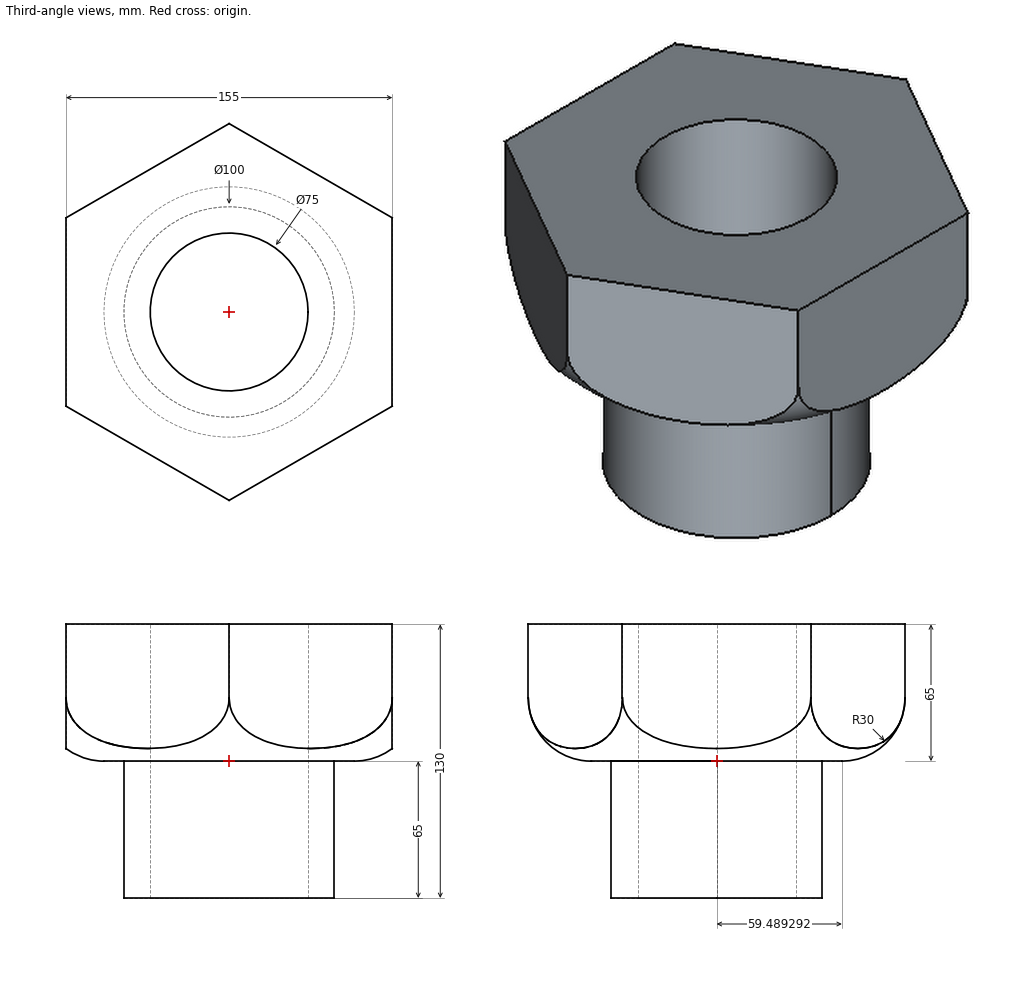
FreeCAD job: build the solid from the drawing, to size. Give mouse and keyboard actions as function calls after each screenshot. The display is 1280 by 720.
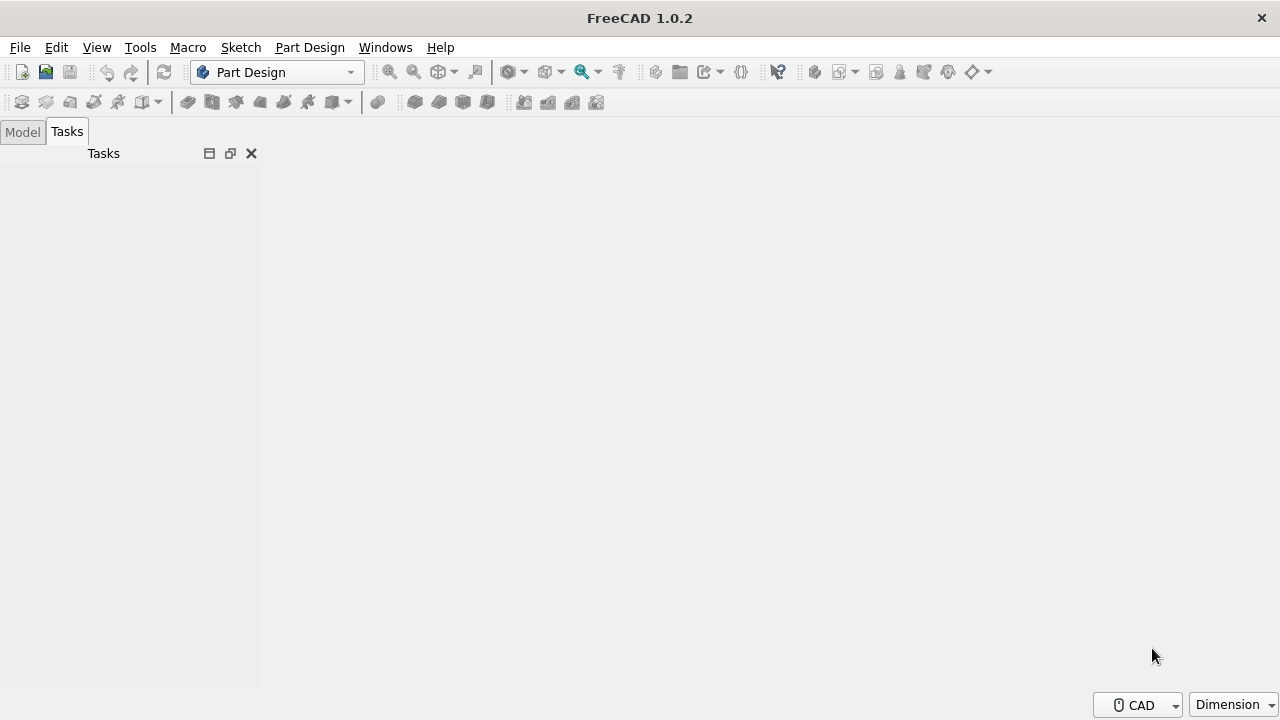
key(ctrl+n)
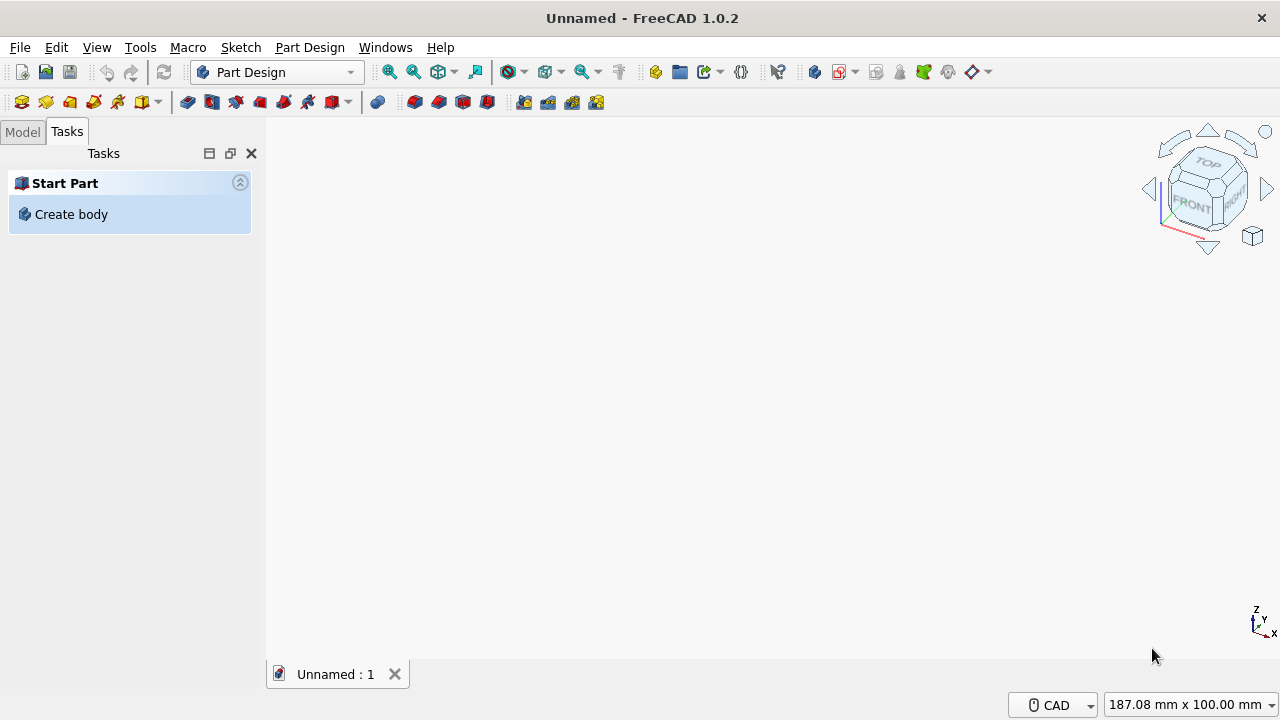
click(840, 72)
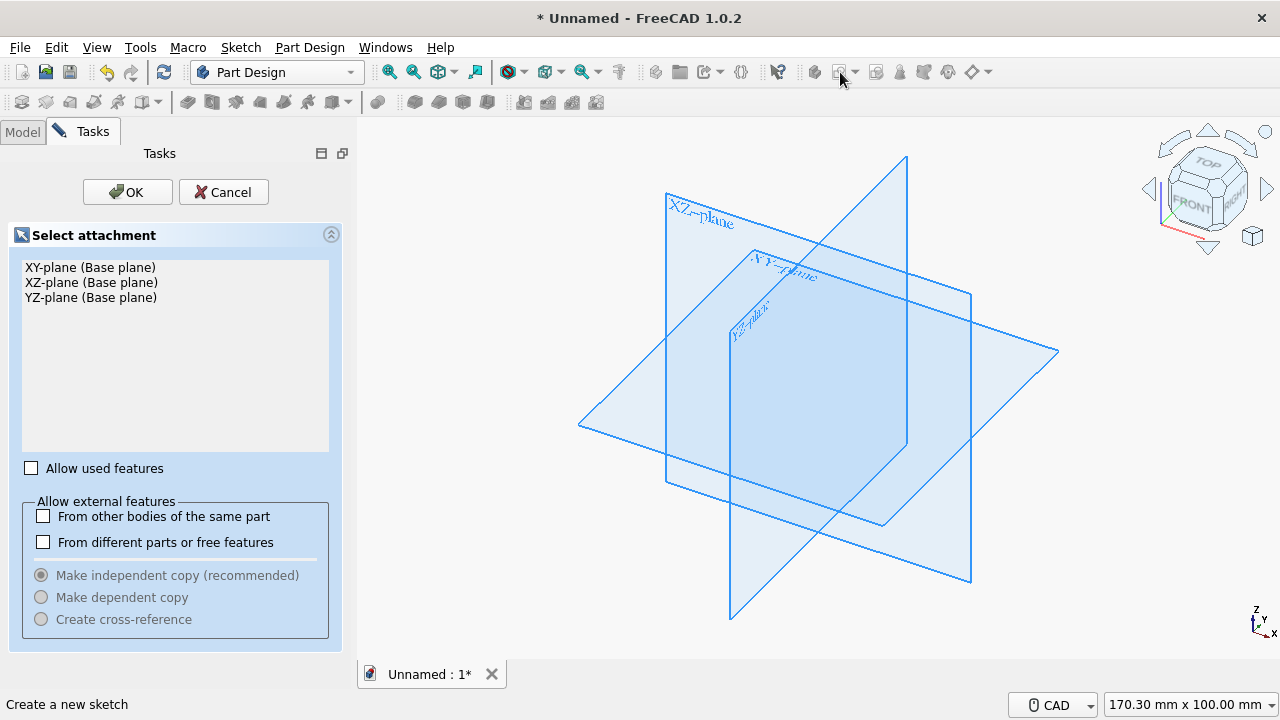
click(82, 268)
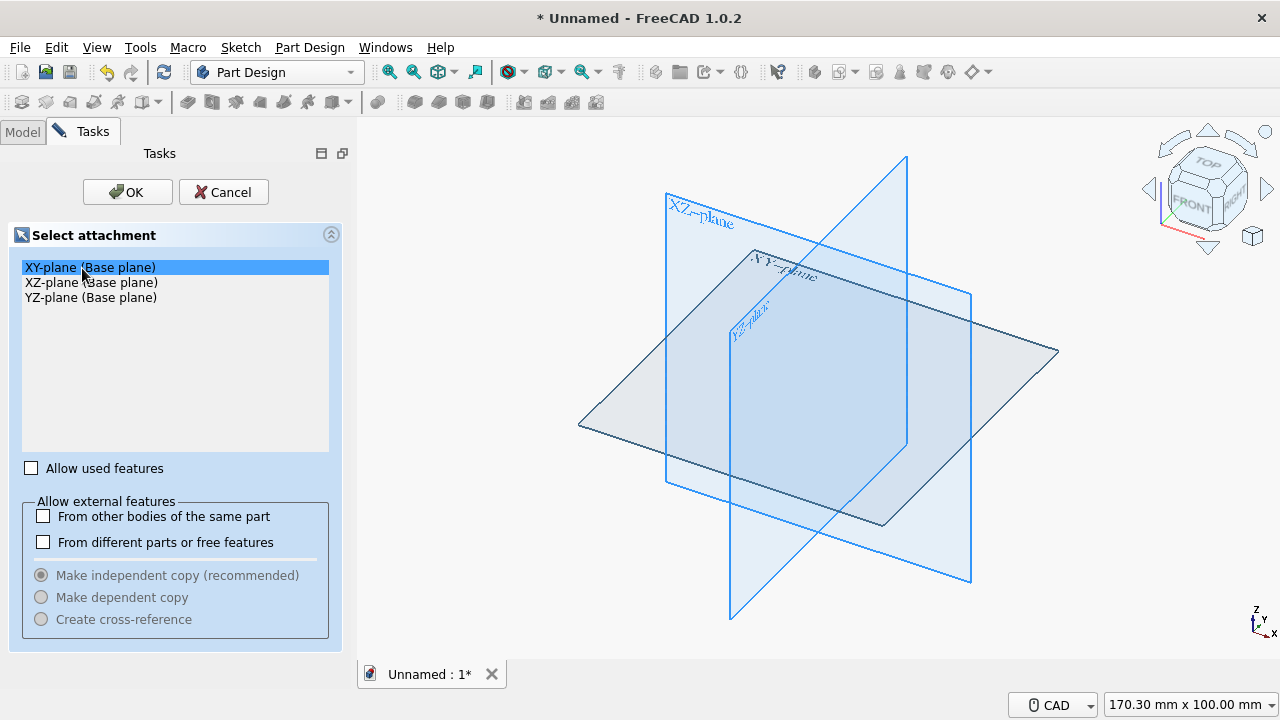
click(128, 192)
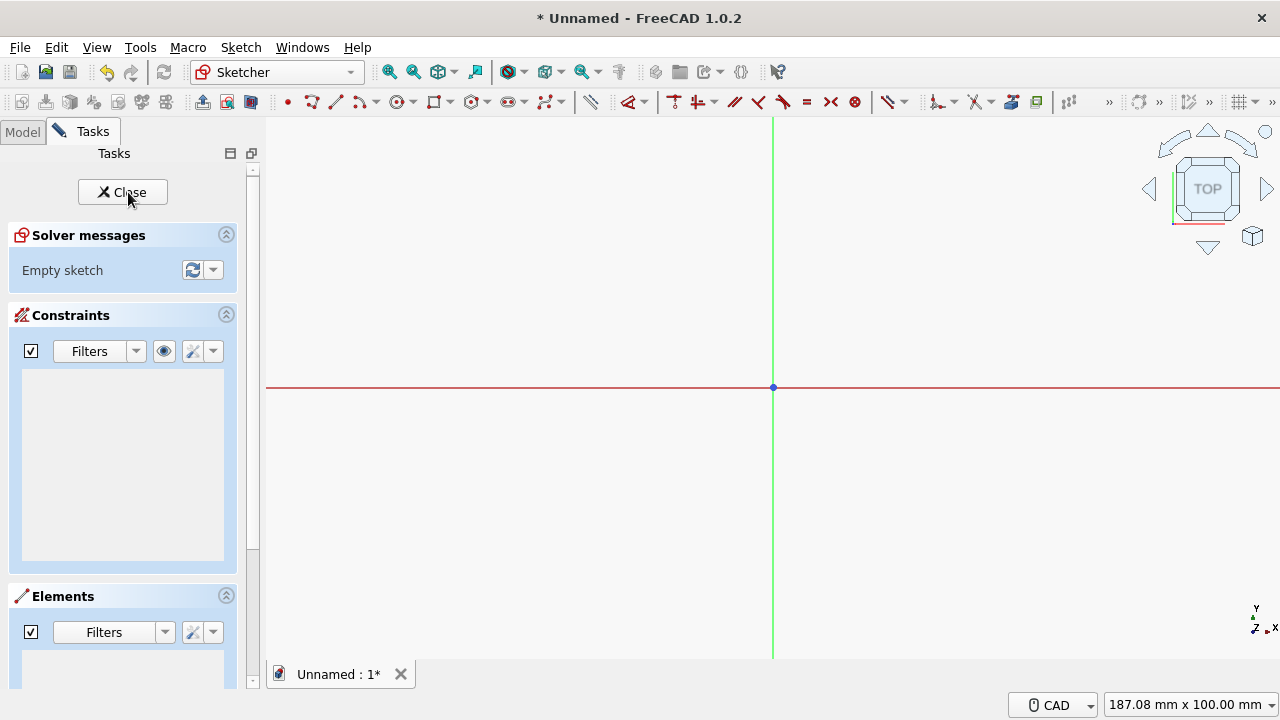
scroll(665, 388, down, 5)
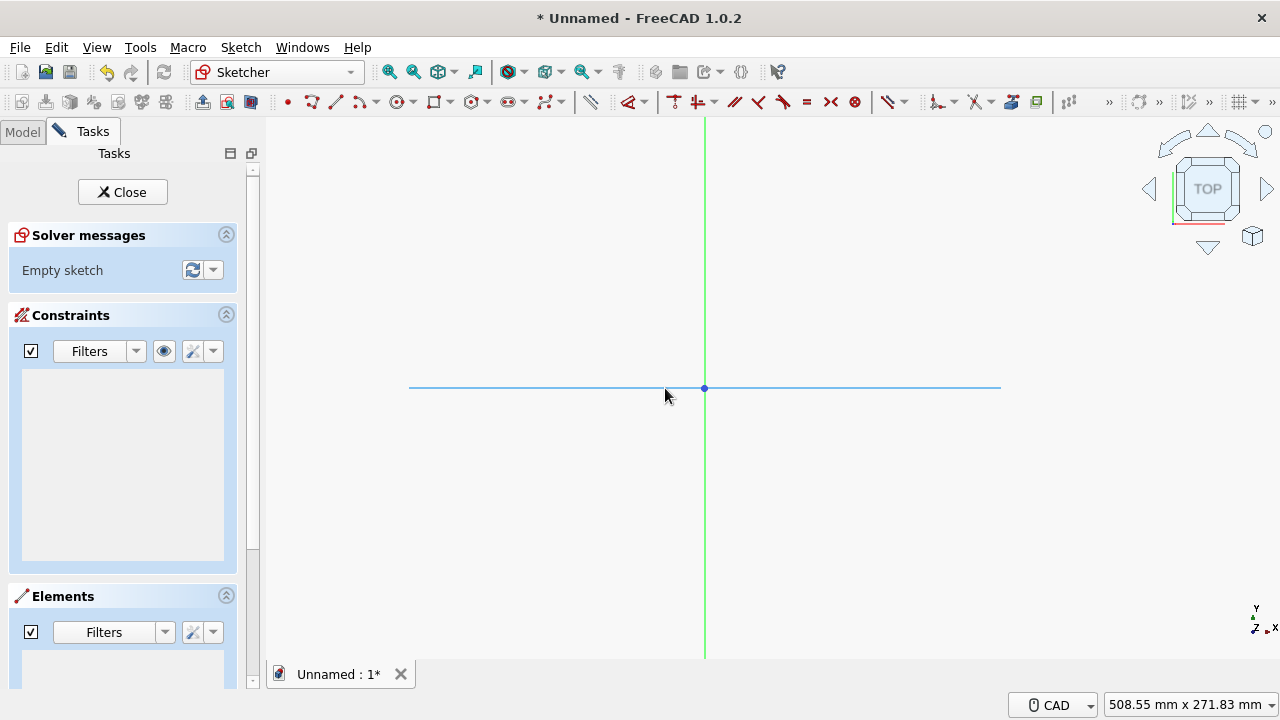
key(g)
key(p)
key(6)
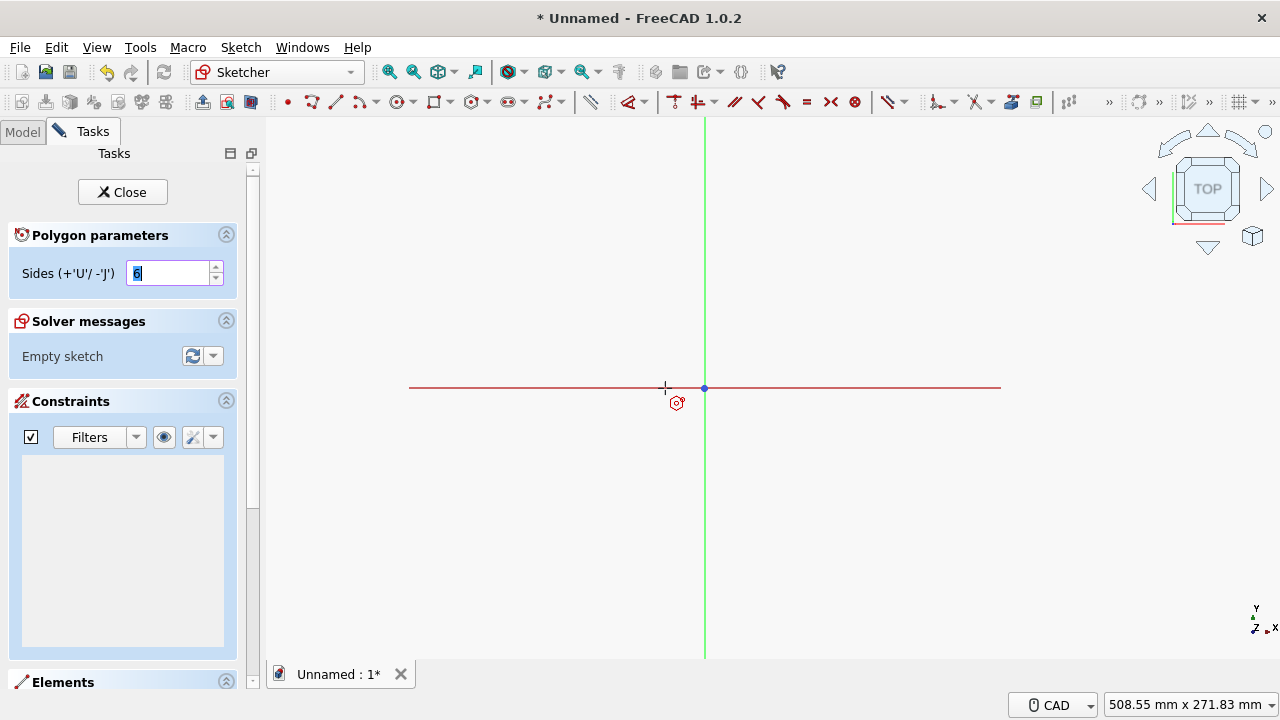
click(705, 388)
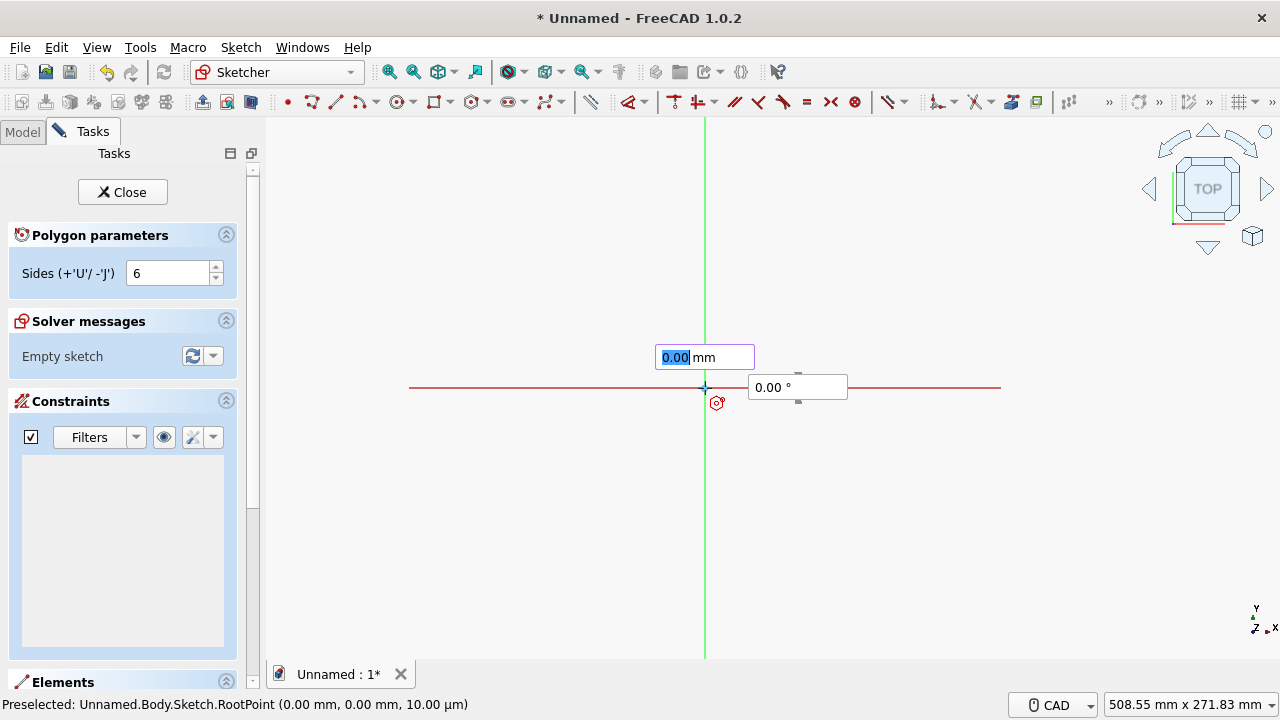
click(705, 210)
right_click(705, 210)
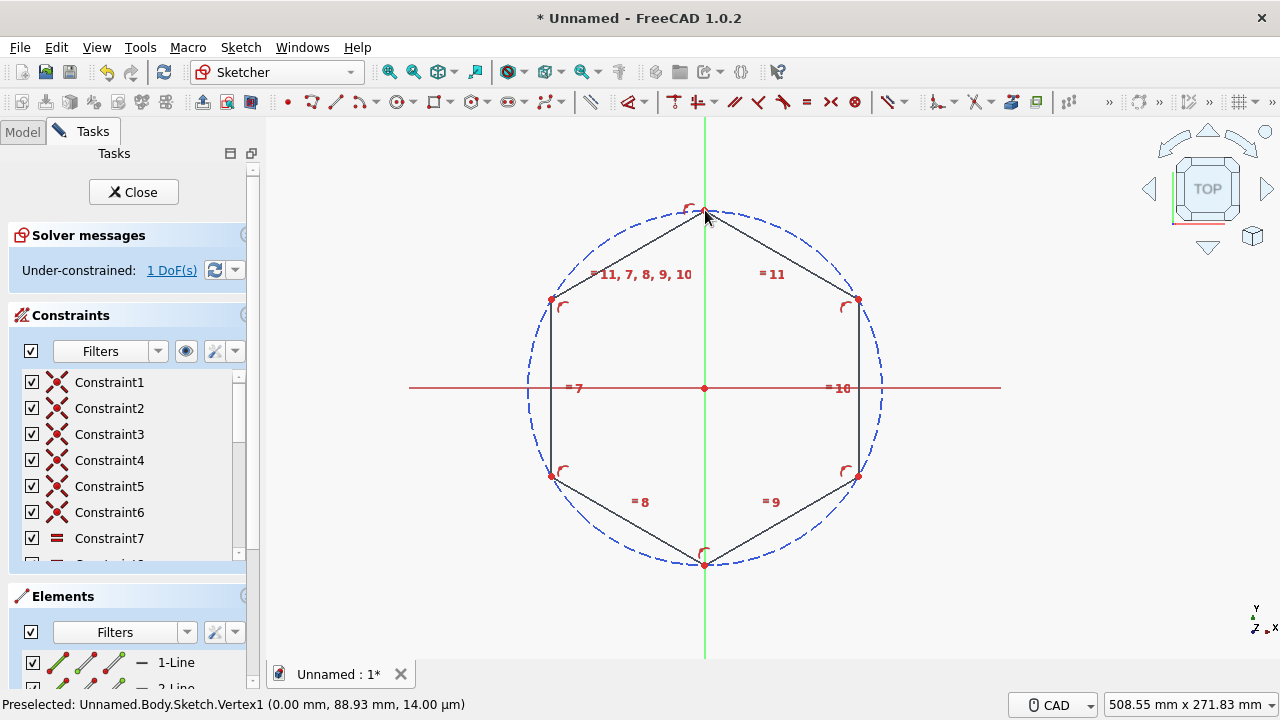
click(551, 300)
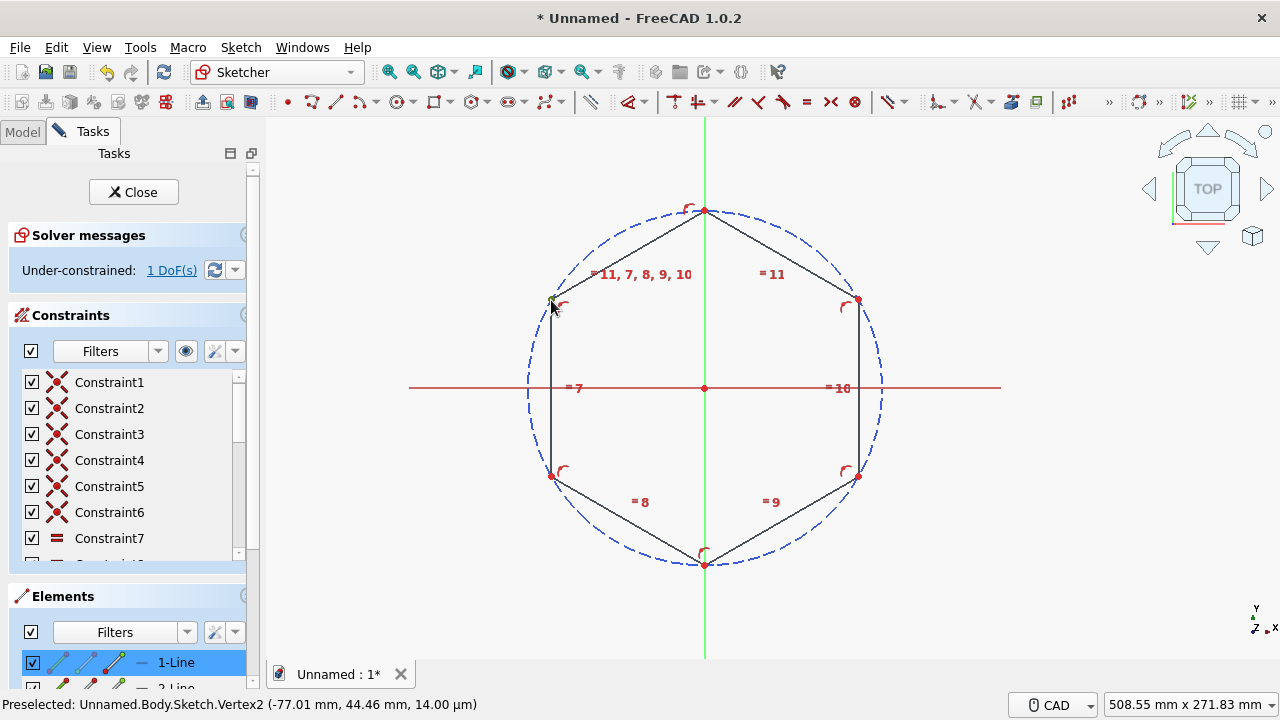
click(859, 477)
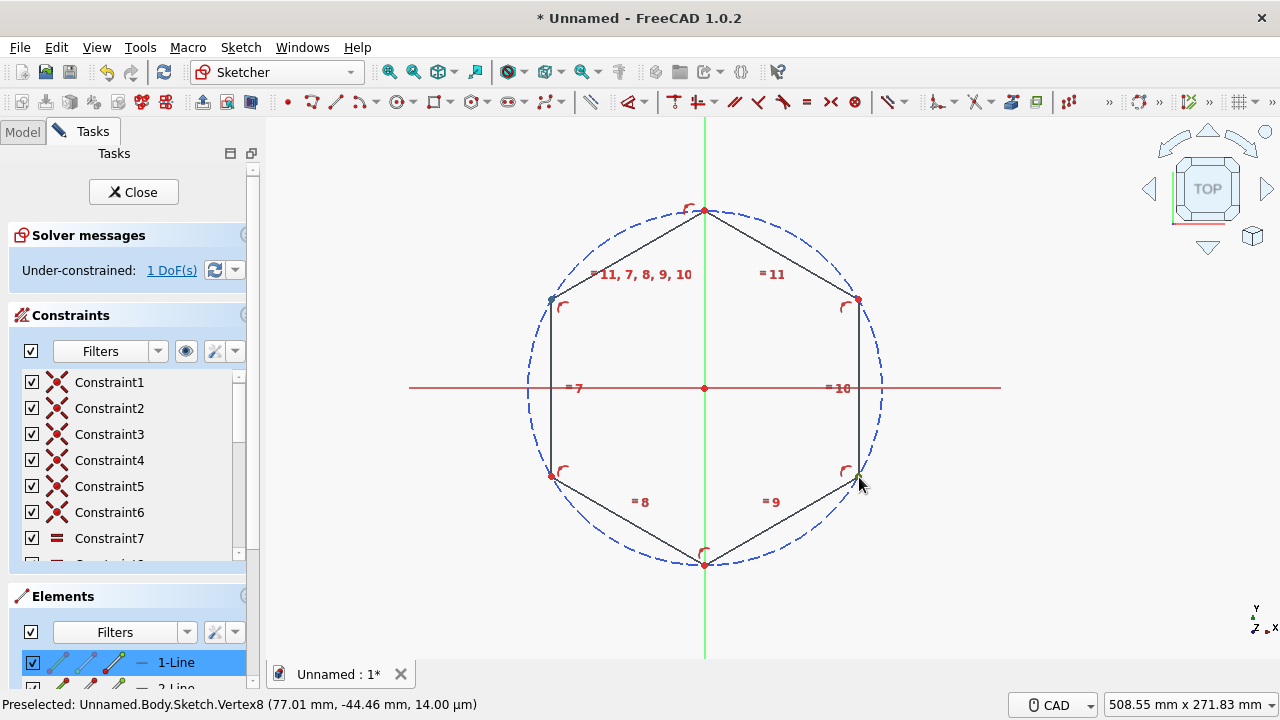
key(l)